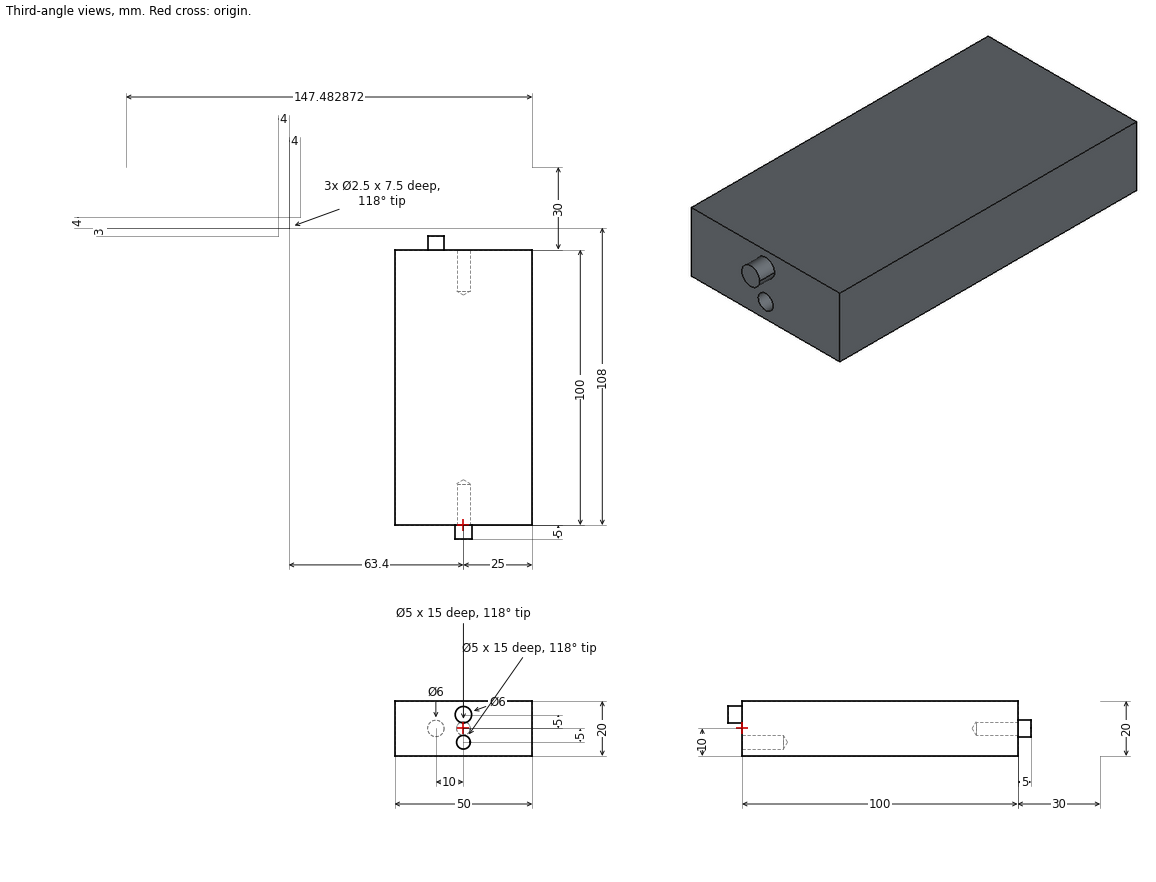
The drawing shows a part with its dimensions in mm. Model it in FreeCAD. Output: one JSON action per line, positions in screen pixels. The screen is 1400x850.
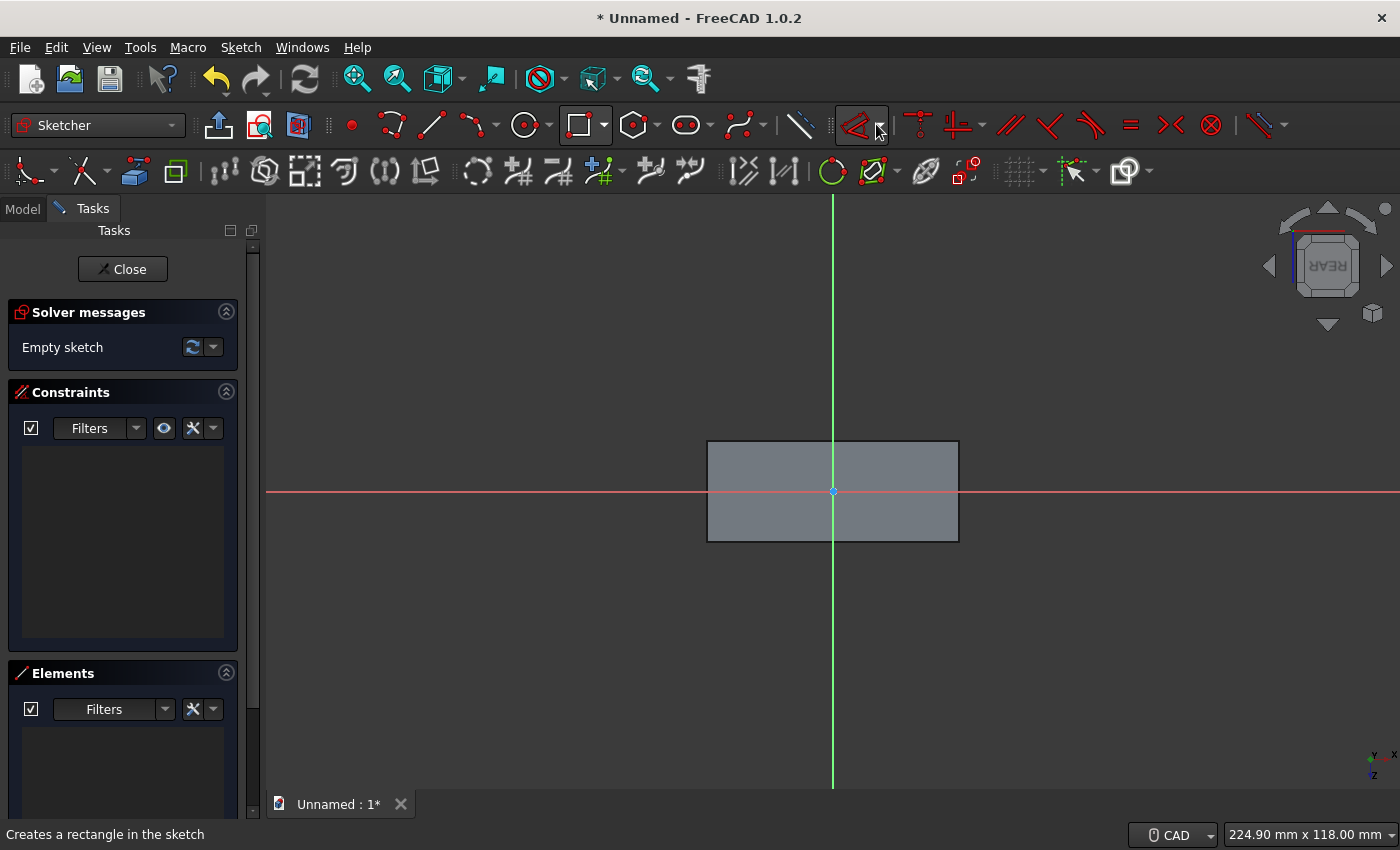
{"action": "scroll", "coordinate": [804, 491], "scroll_direction": "up", "scroll_amount": 12}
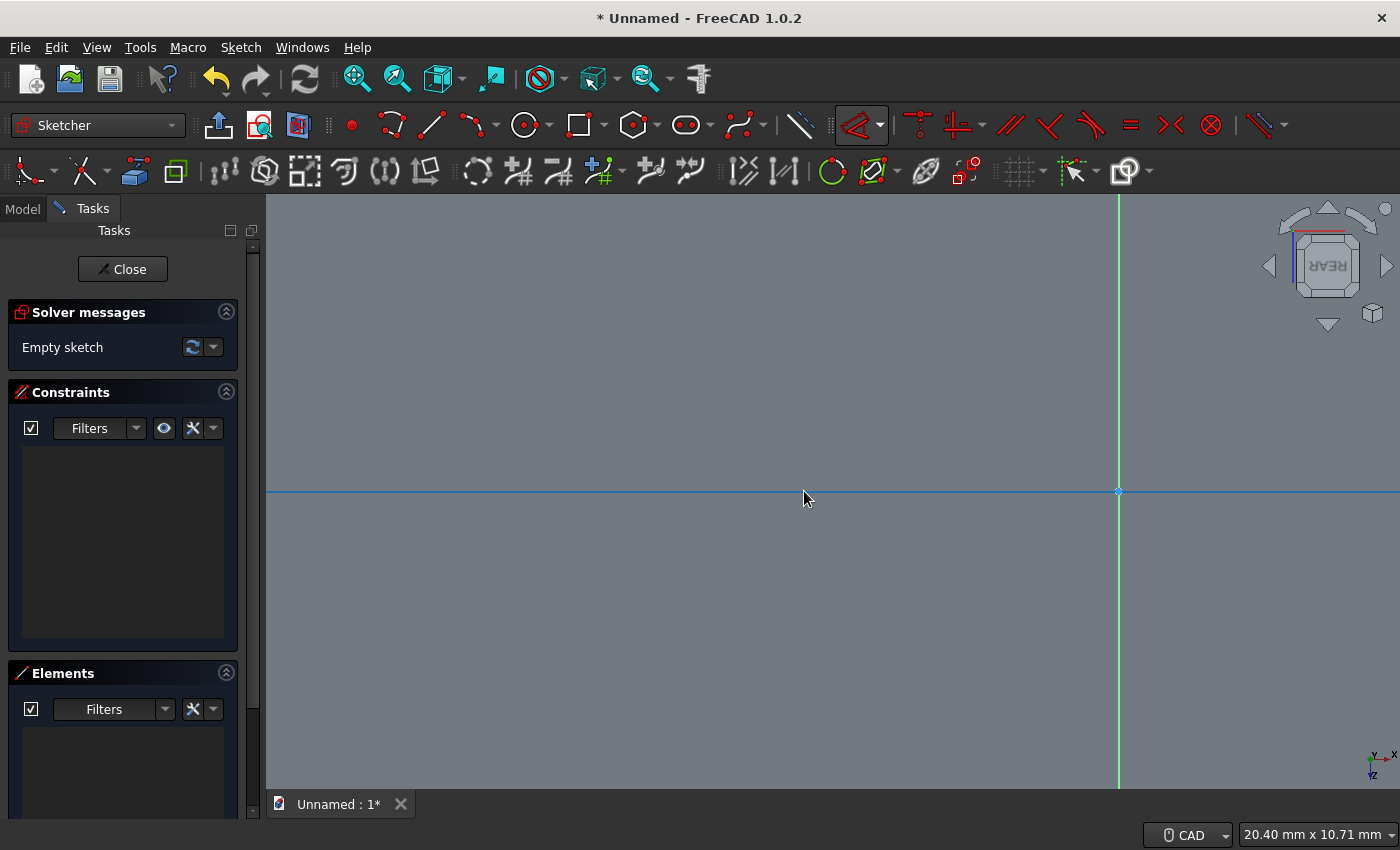
{"action": "key", "text": "g c"}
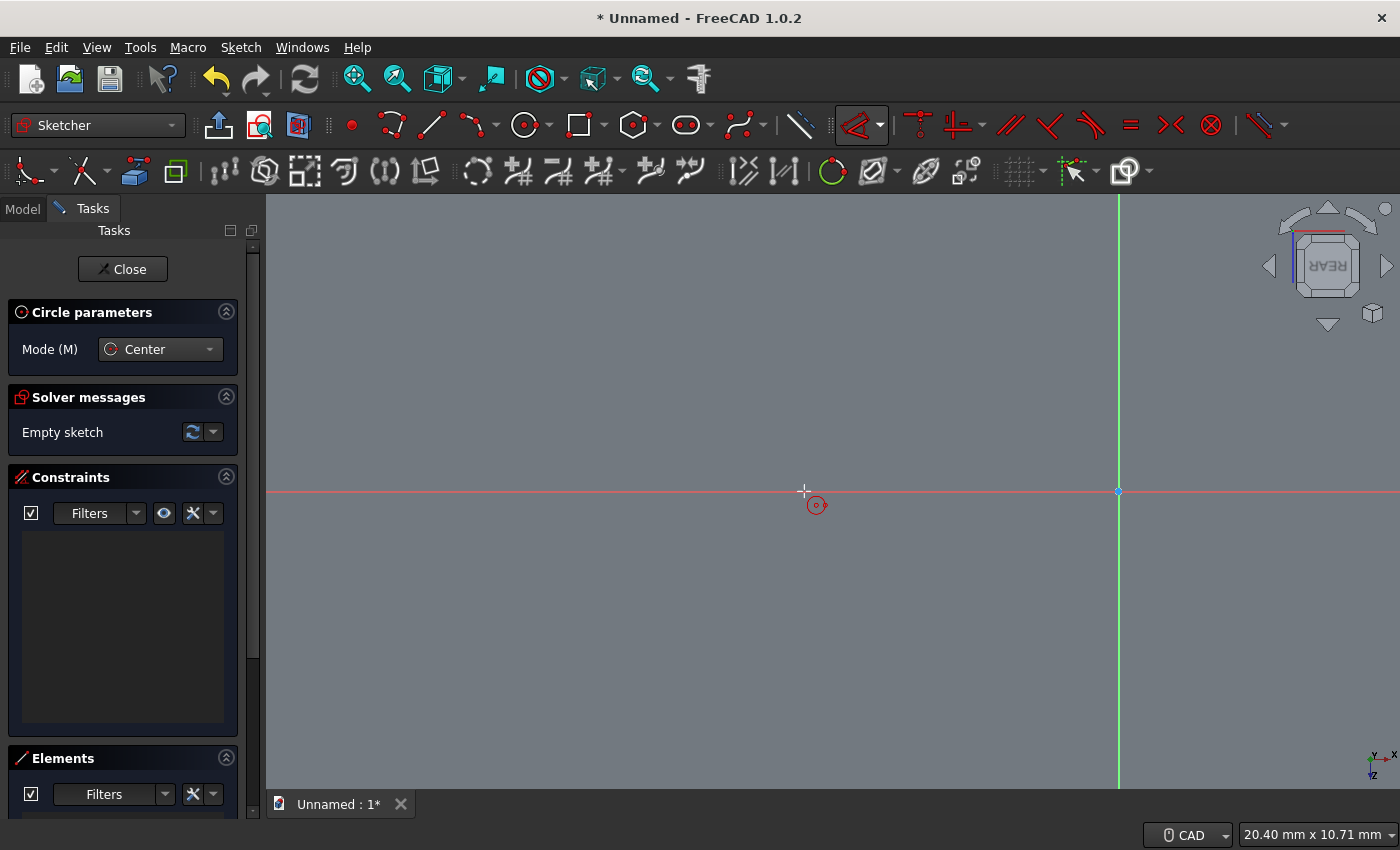
{"action": "left_click", "coordinate": [563, 491]}
{"action": "left_click", "coordinate": [681, 374]}
{"action": "key", "text": "Escape"}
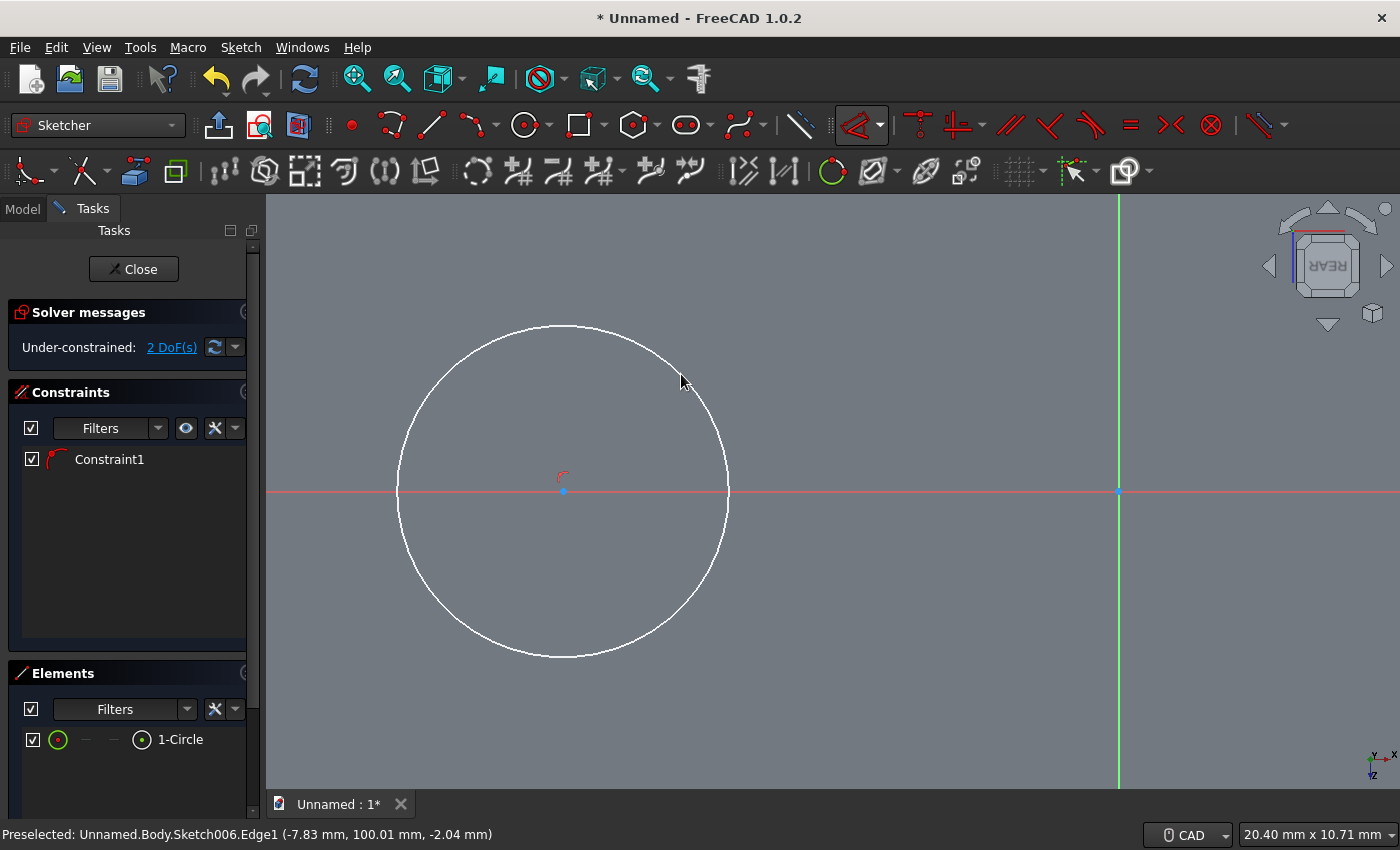
{"action": "left_click", "coordinate": [680, 374]}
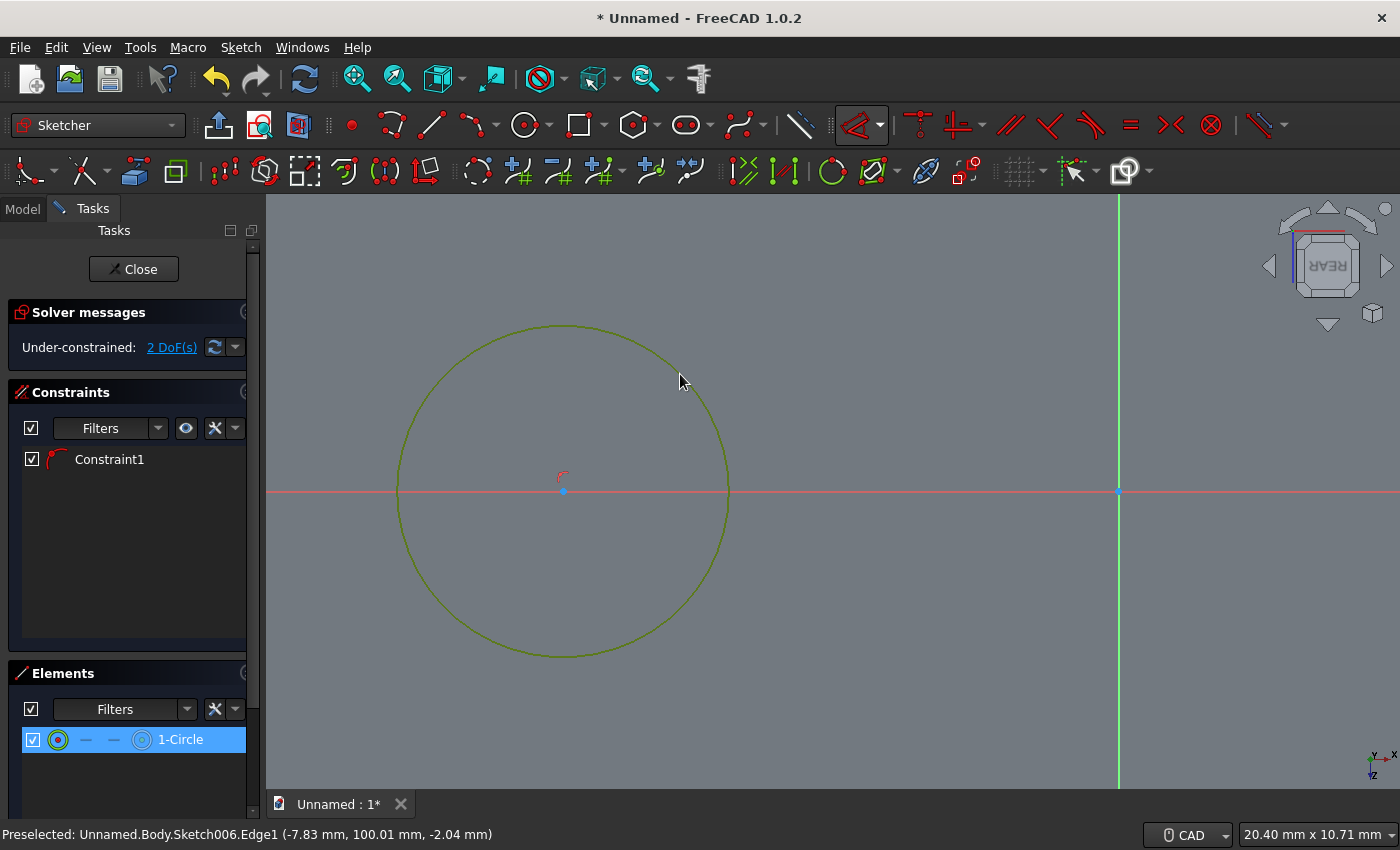
{"action": "left_click", "coordinate": [882, 126]}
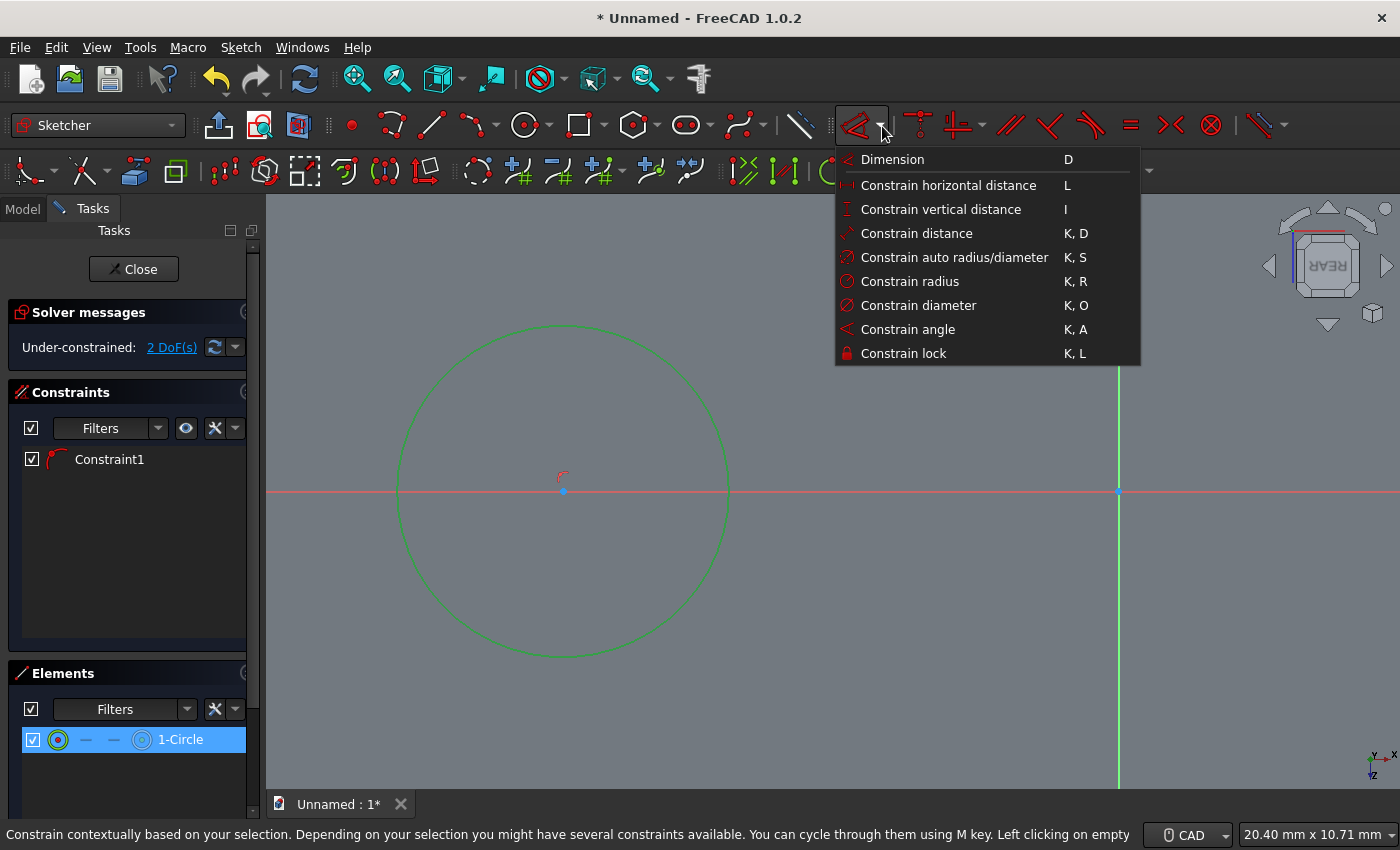
{"action": "left_click", "coordinate": [988, 305]}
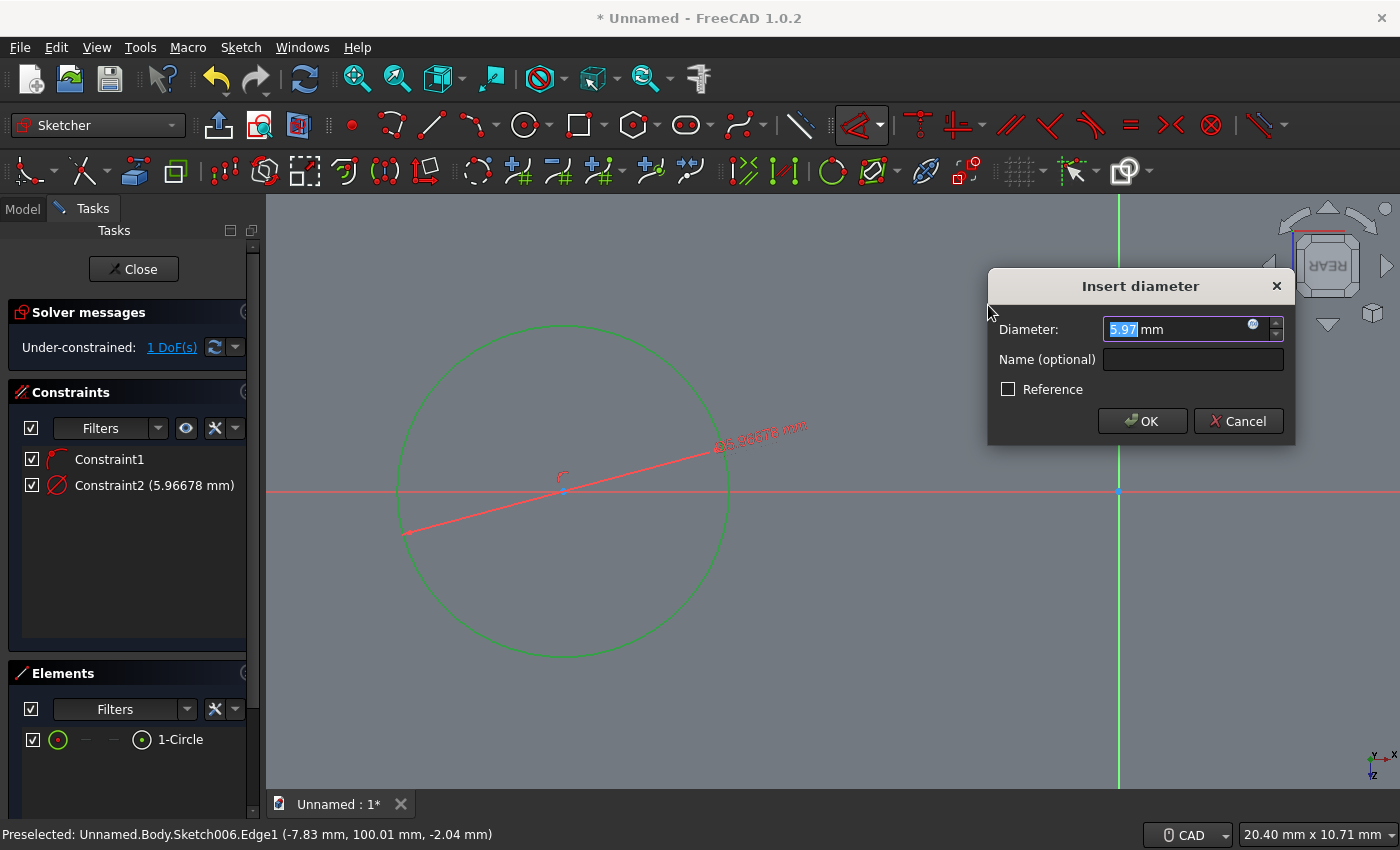
{"action": "type", "text": "6"}
{"action": "key", "text": "Return"}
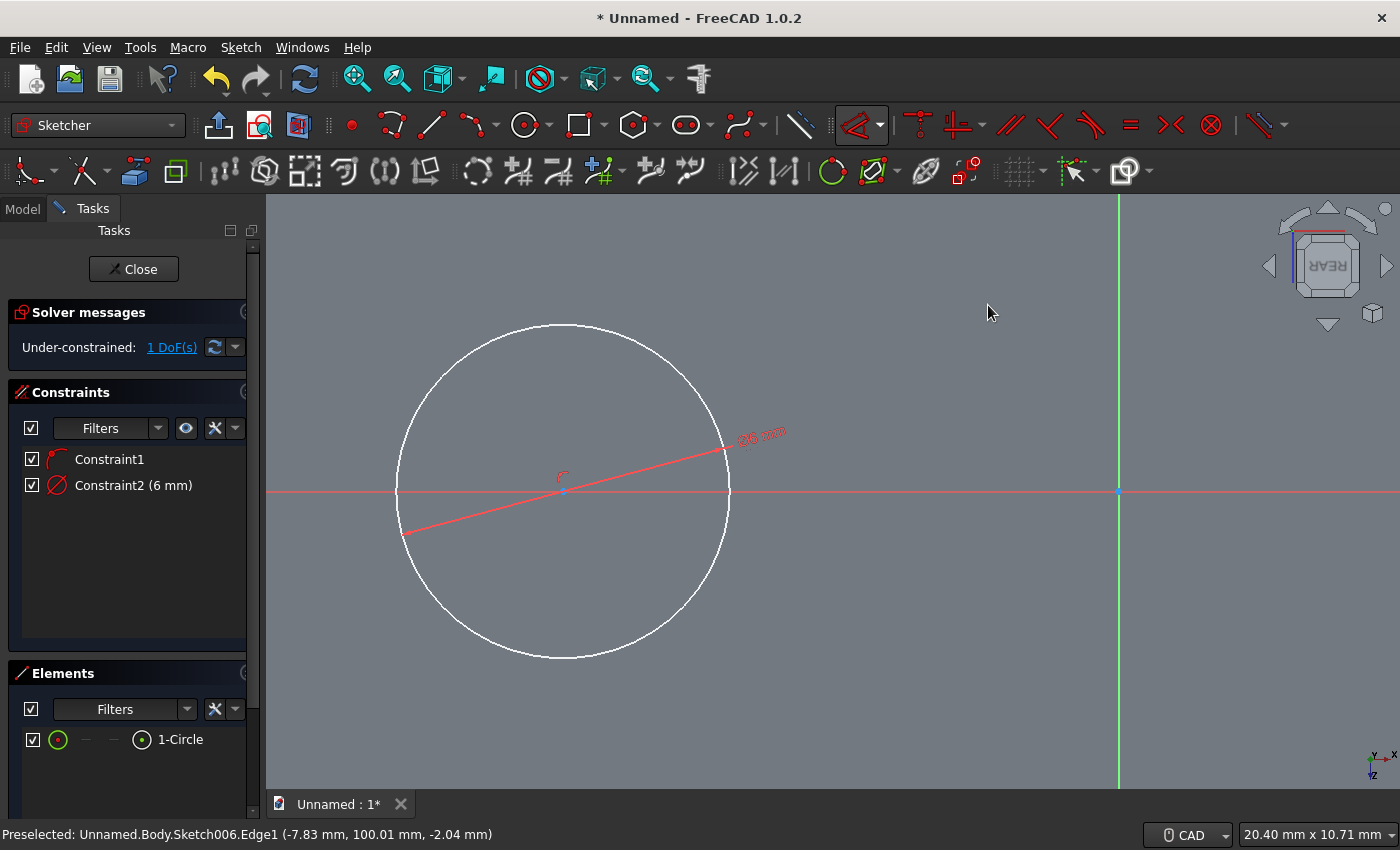
{"action": "left_click", "coordinate": [563, 491]}